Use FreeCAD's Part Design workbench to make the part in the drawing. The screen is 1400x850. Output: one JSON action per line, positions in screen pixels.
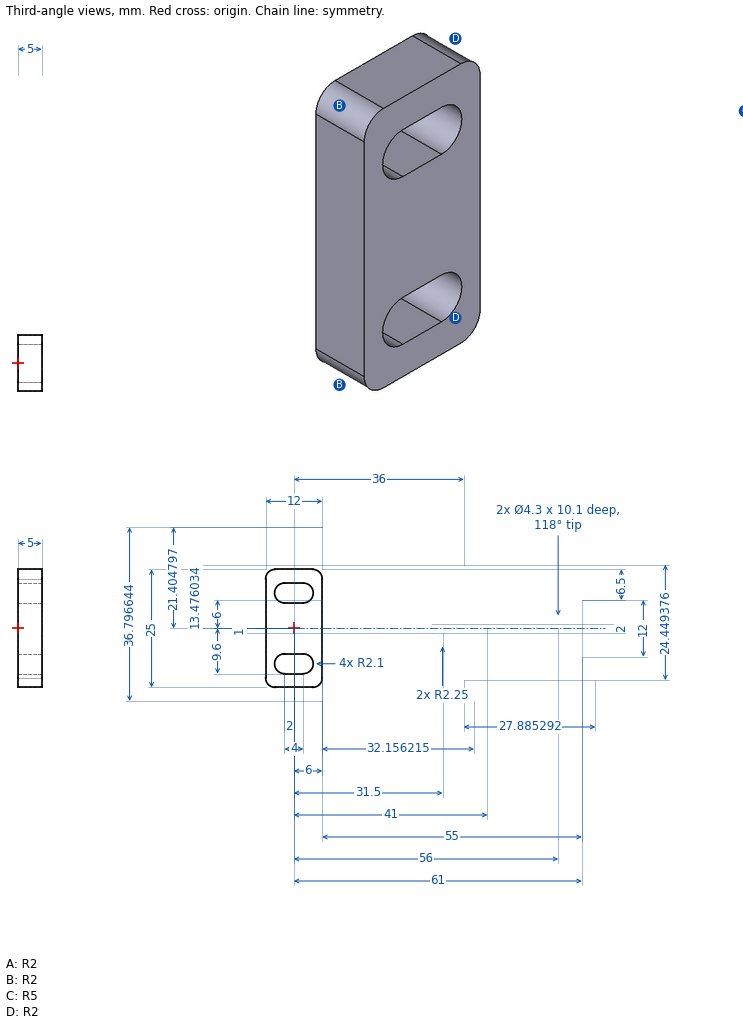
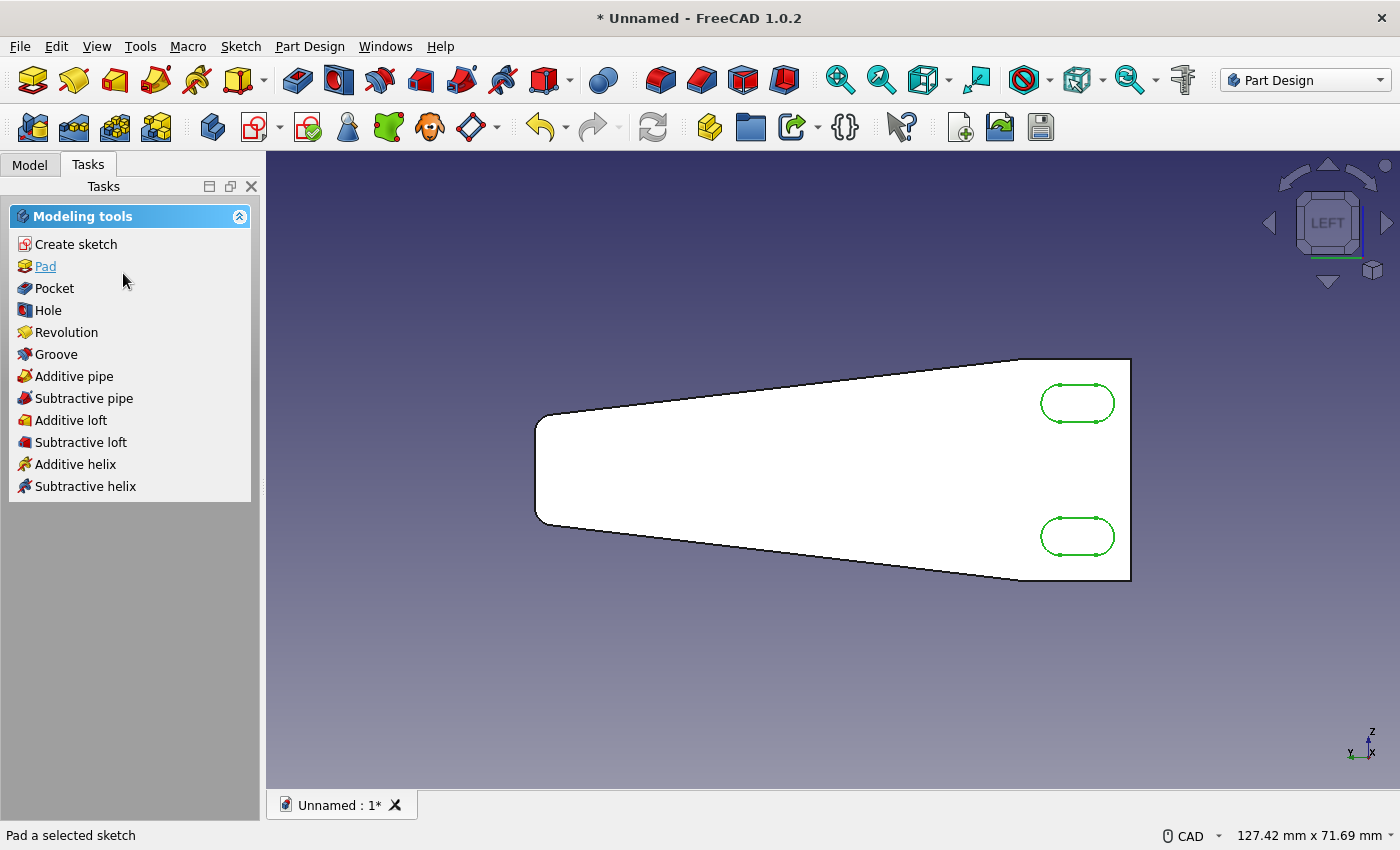
{"action": "left_click", "coordinate": [298, 80]}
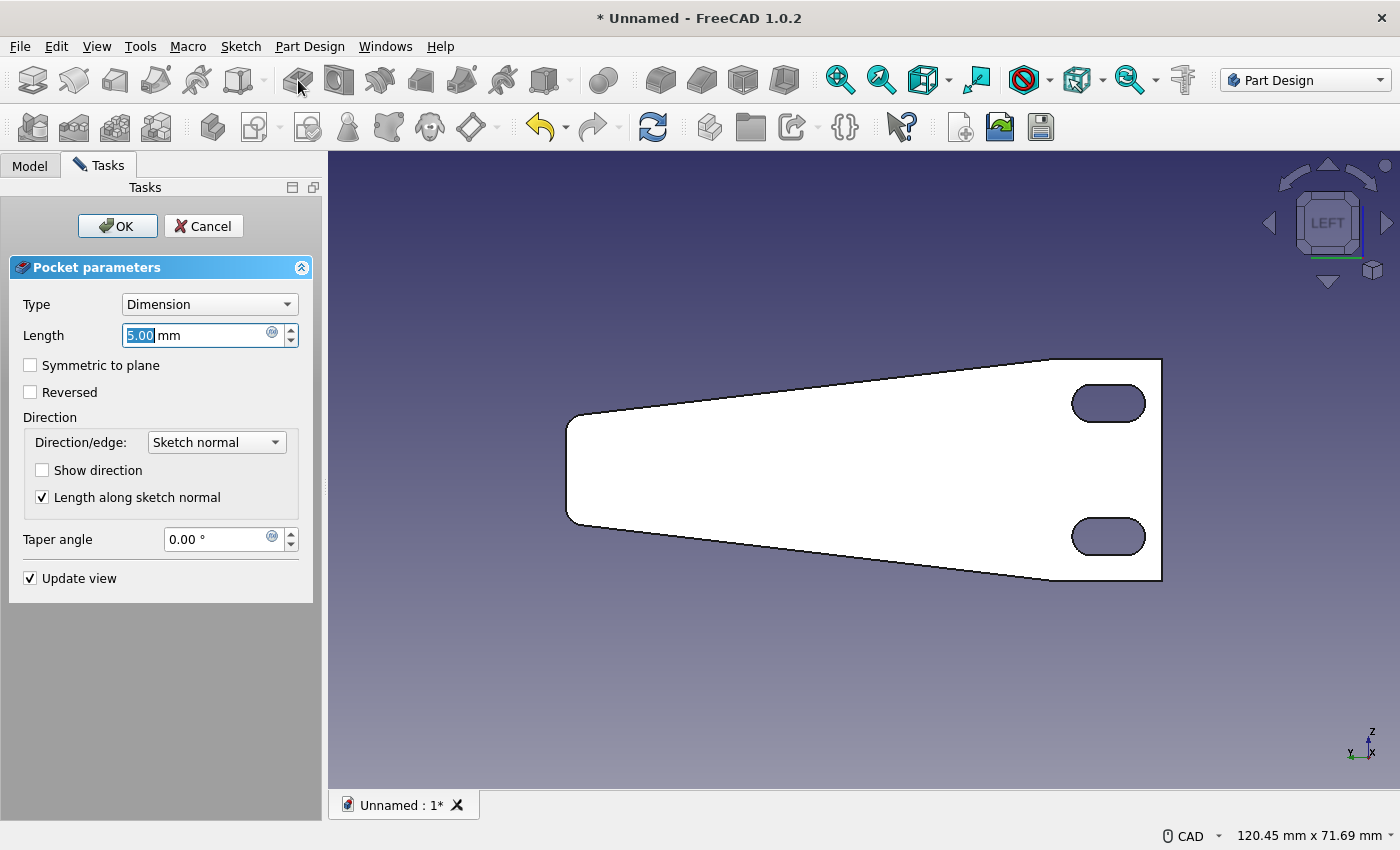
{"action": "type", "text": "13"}
{"action": "key", "text": "Tab"}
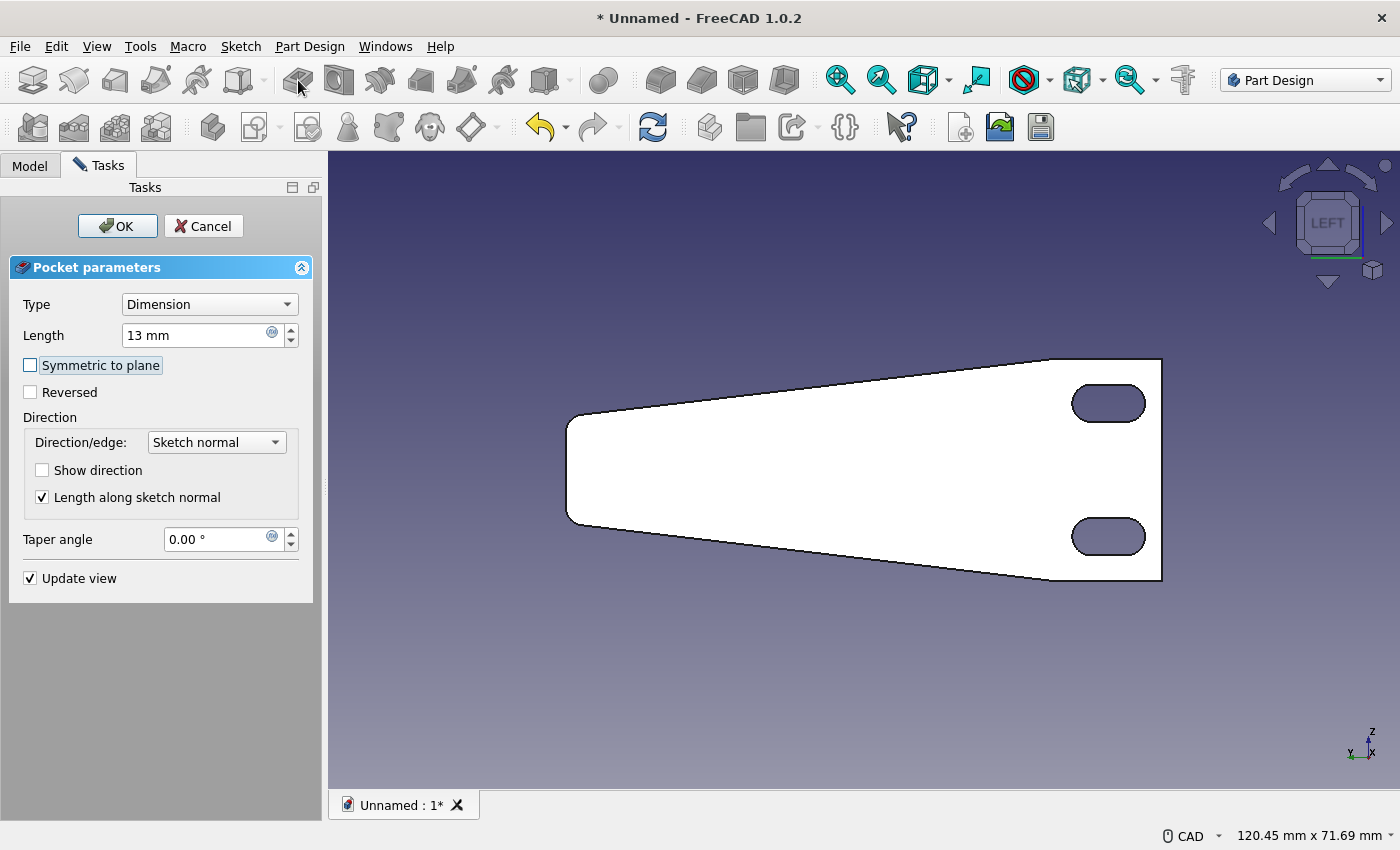
{"action": "left_click", "coordinate": [118, 226]}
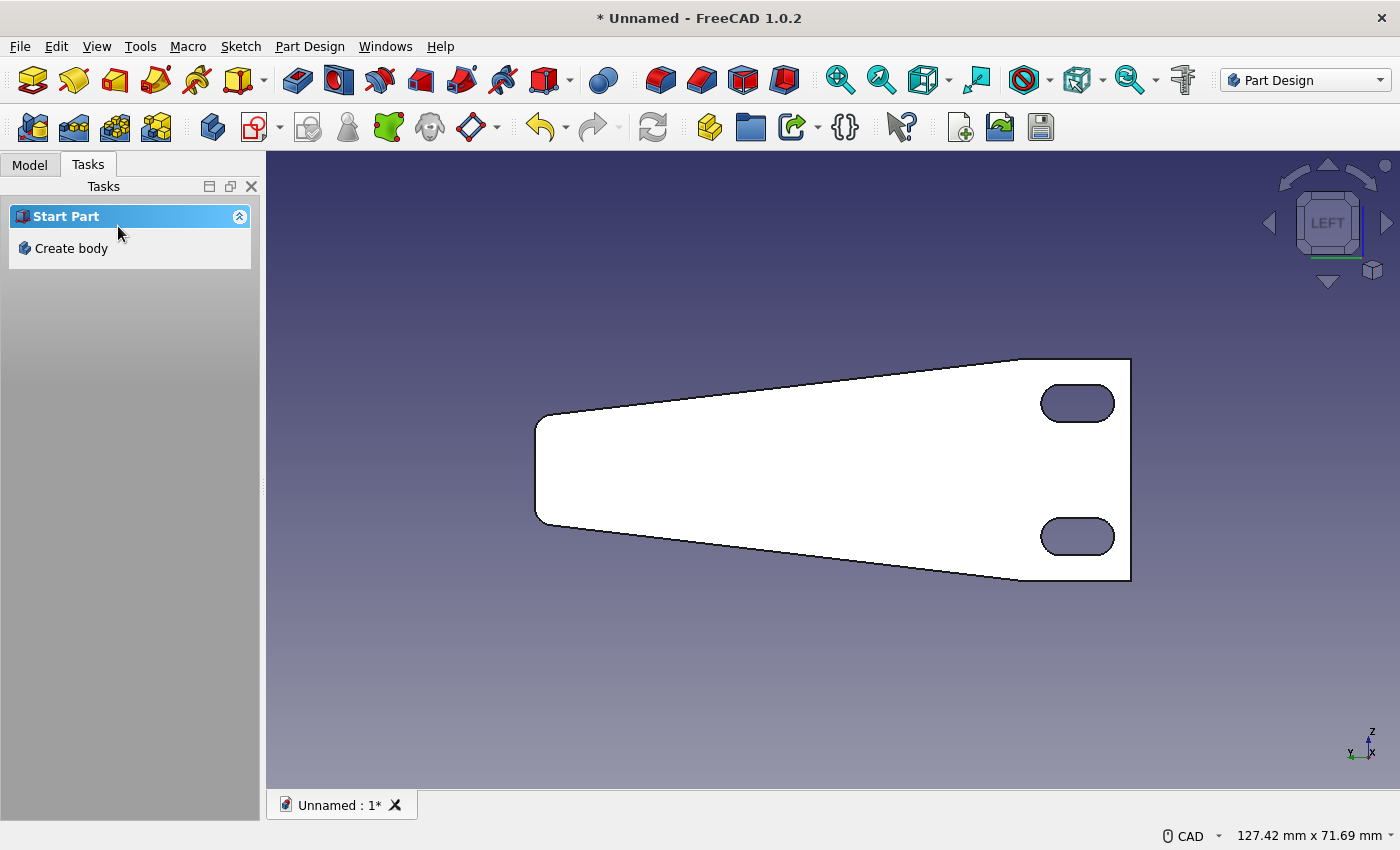
{"action": "key", "text": "0"}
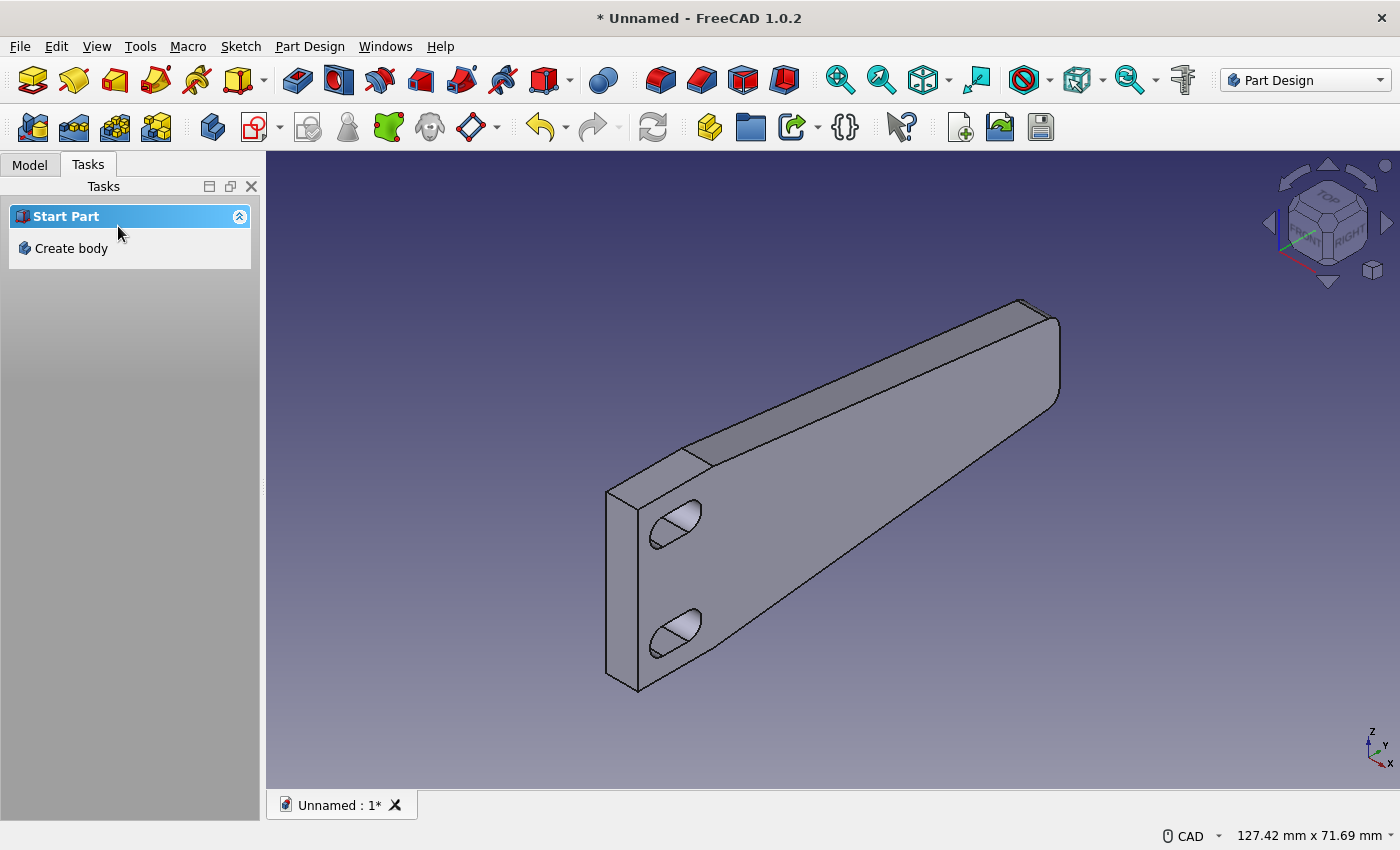
{"action": "left_click", "coordinate": [622, 500]}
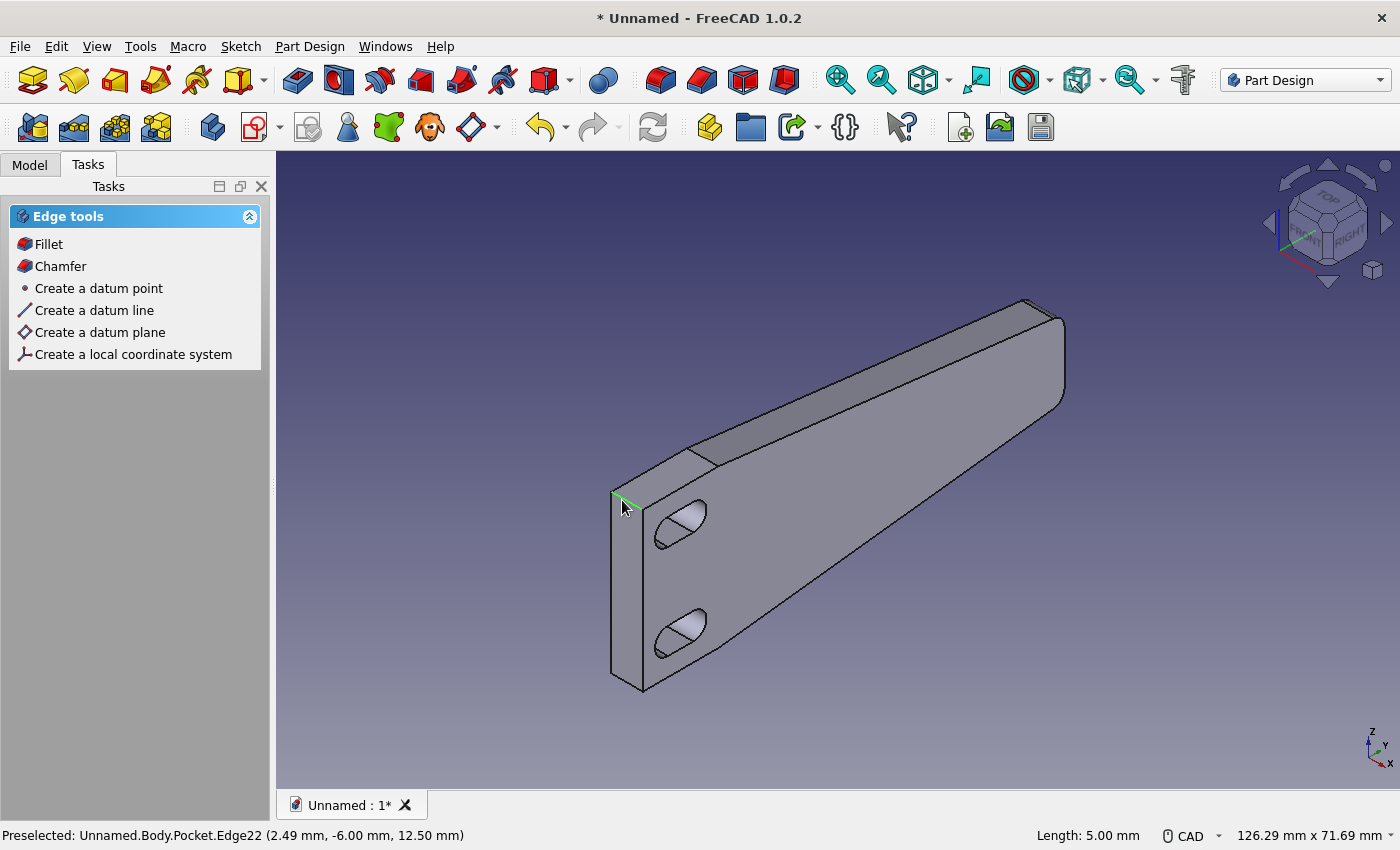
{"action": "key", "text": "2"}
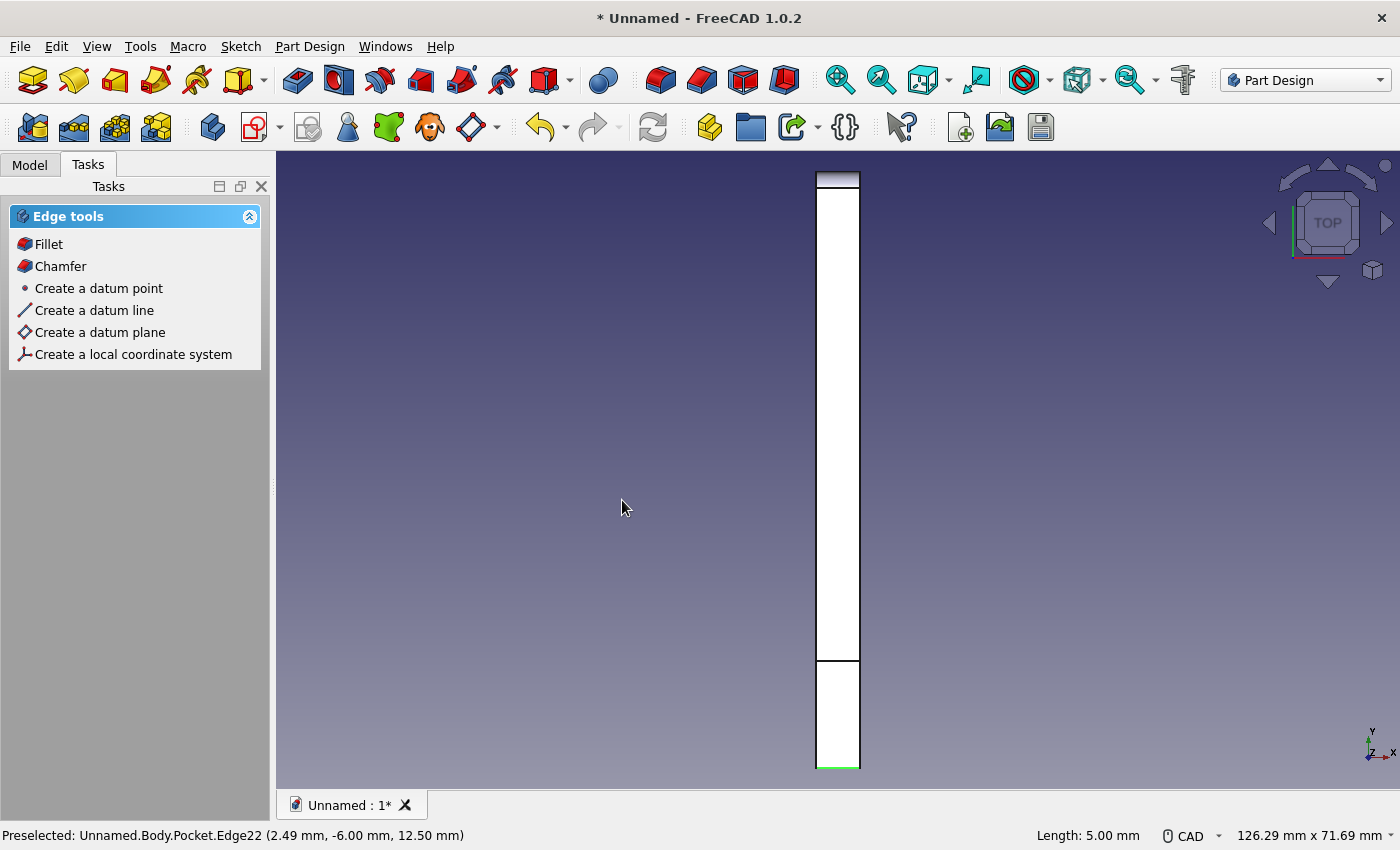
{"action": "key", "text": "1"}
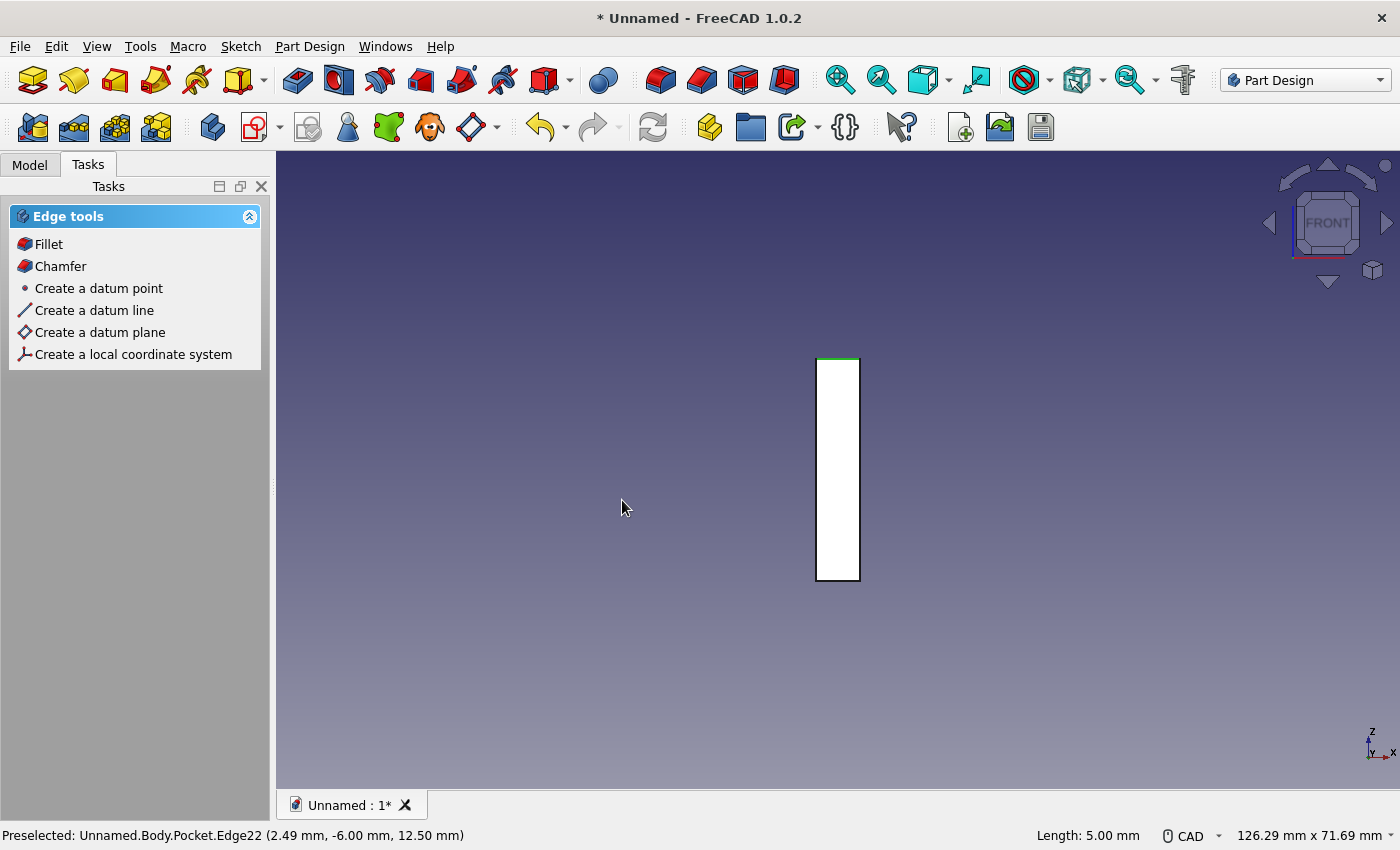
{"action": "left_click", "coordinate": [841, 80]}